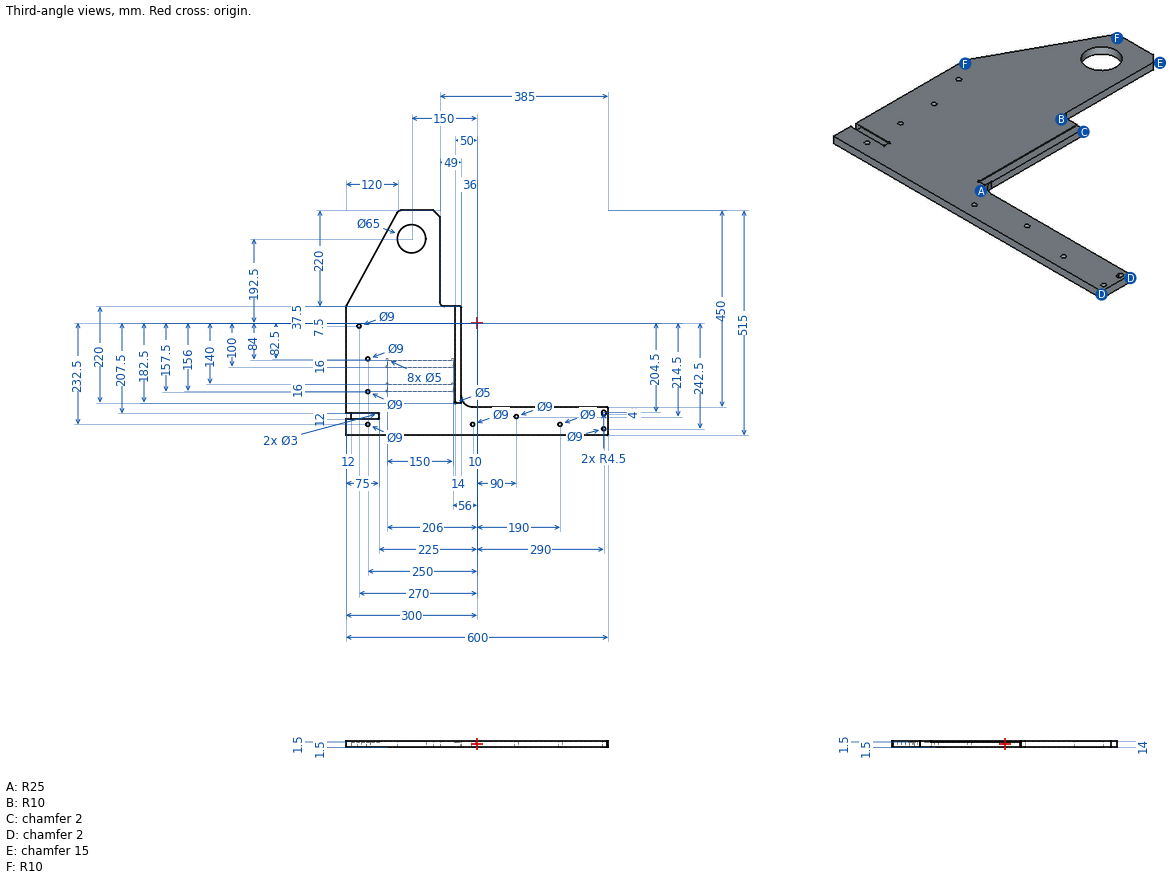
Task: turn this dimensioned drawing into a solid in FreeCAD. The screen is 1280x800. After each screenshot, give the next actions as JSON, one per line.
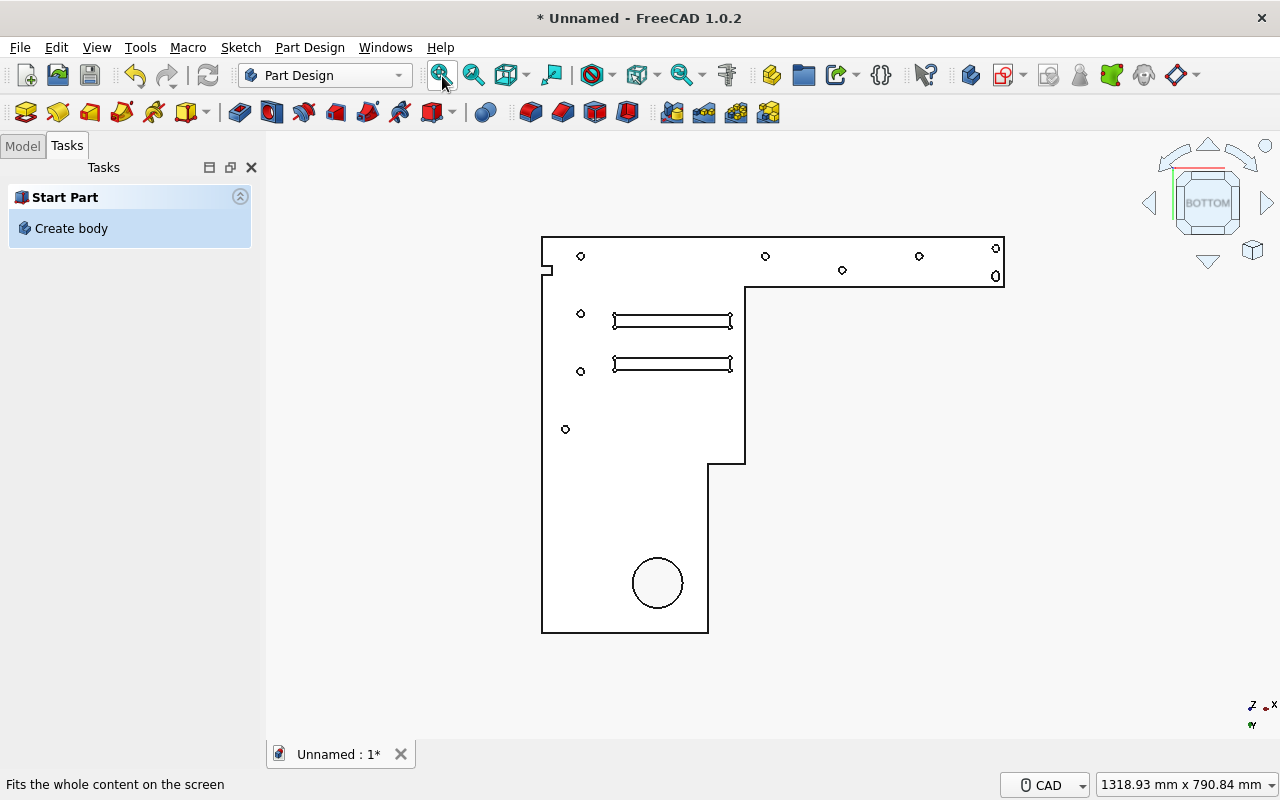
{"action": "key", "text": "4"}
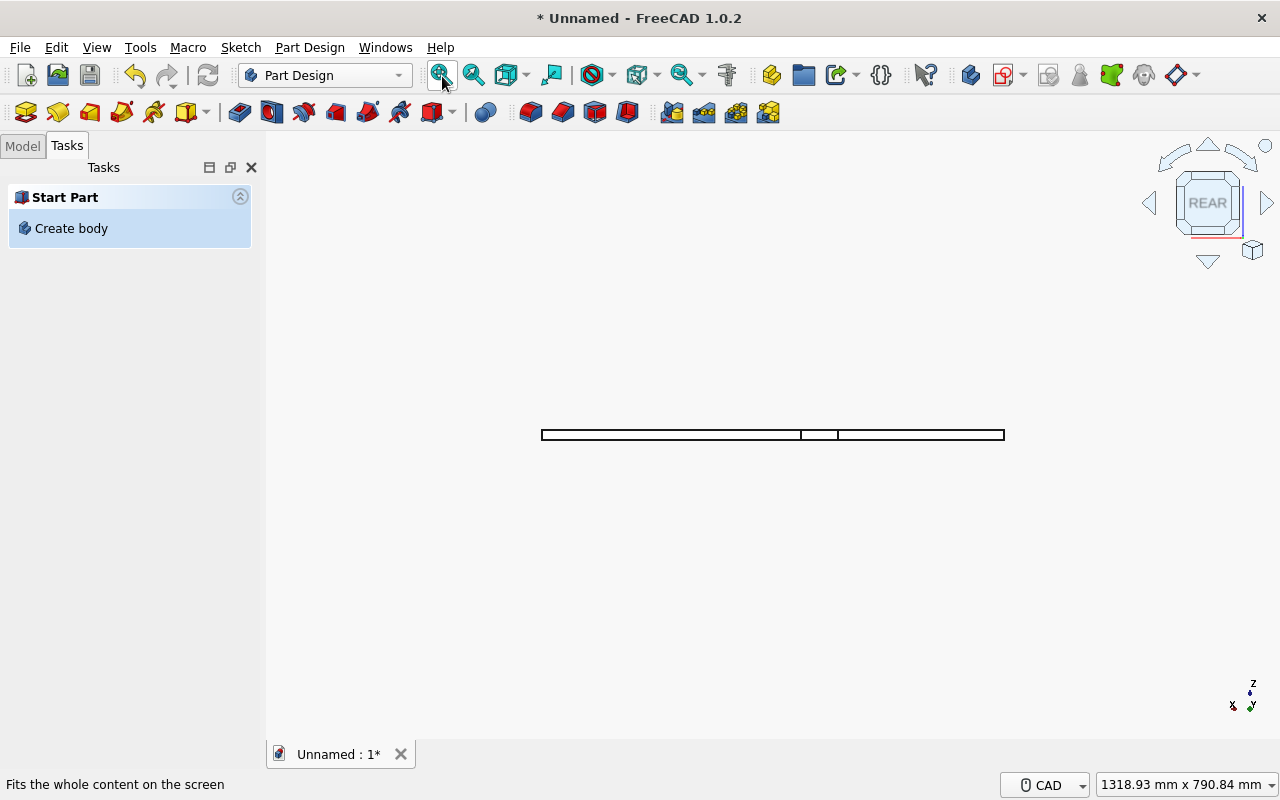
{"action": "scroll", "coordinate": [801, 434], "scroll_direction": "up", "scroll_amount": 7}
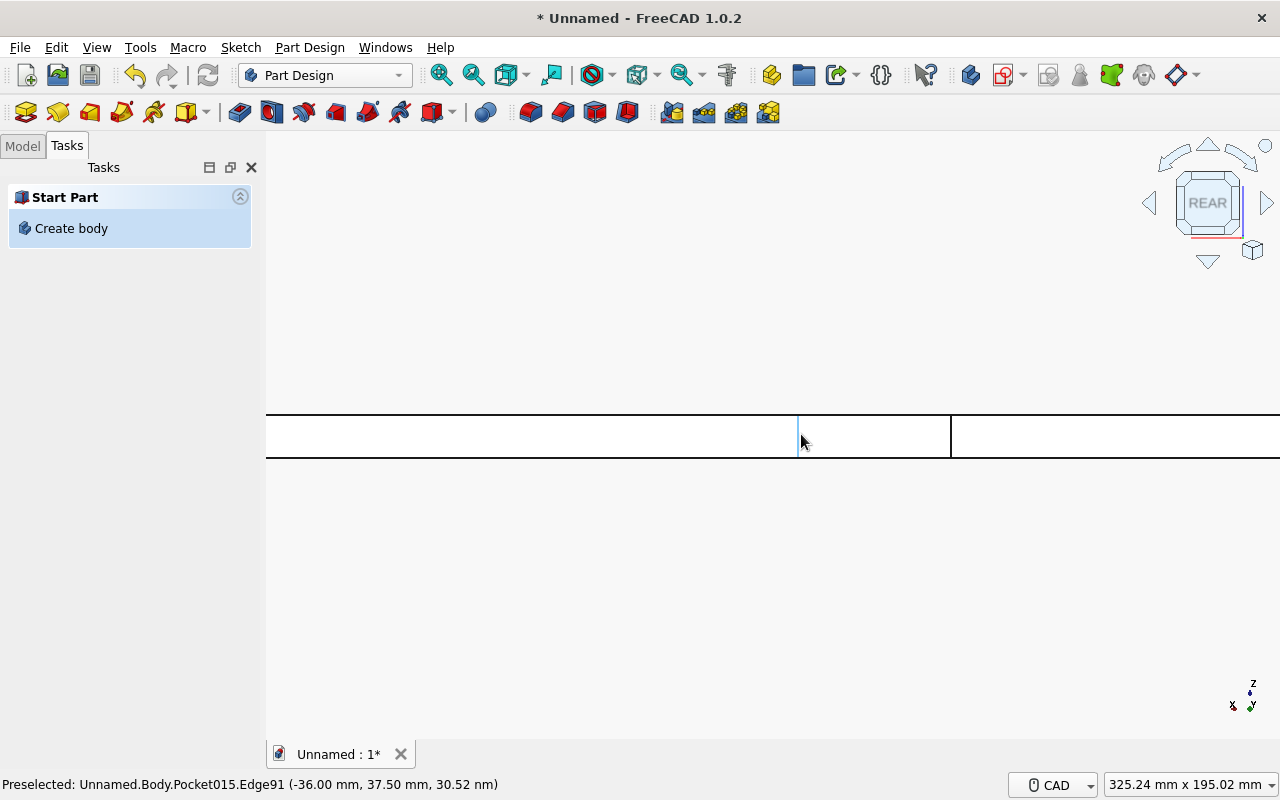
{"action": "left_click", "coordinate": [442, 76]}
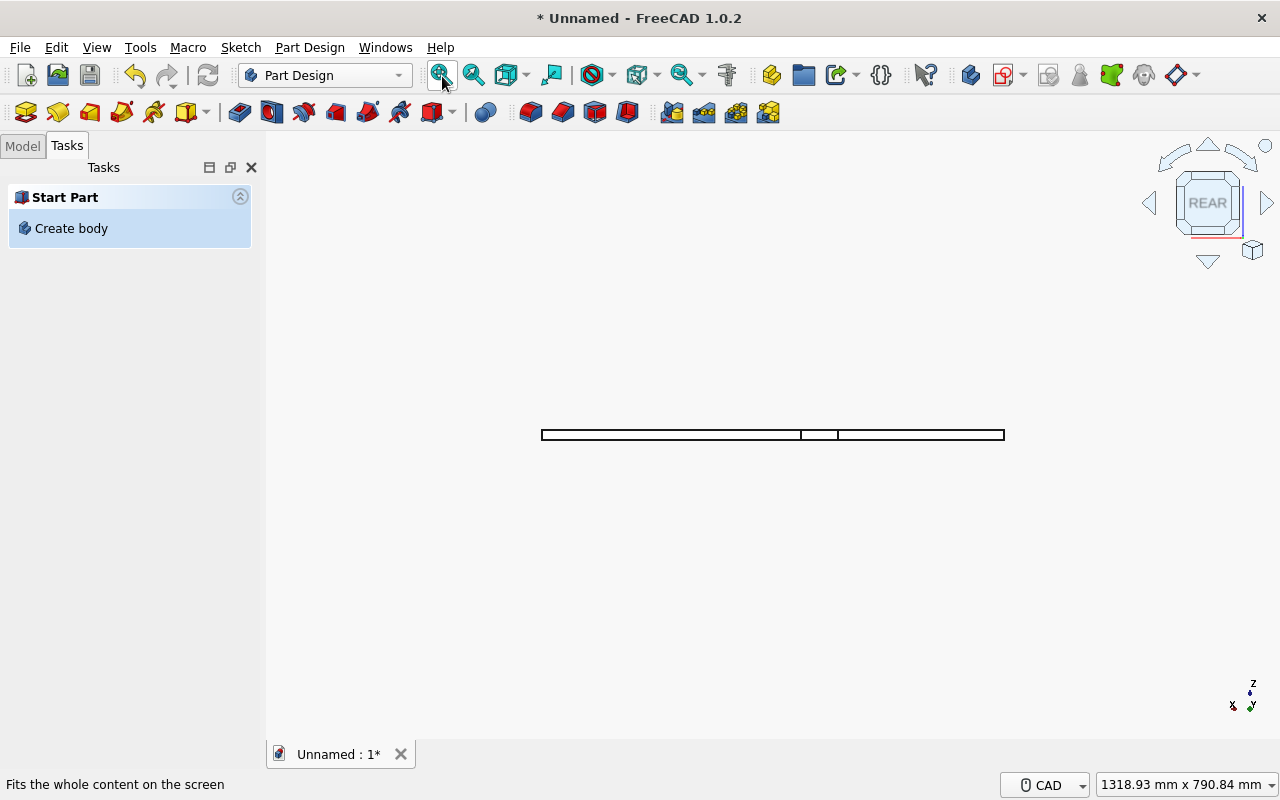
{"action": "key", "text": "6"}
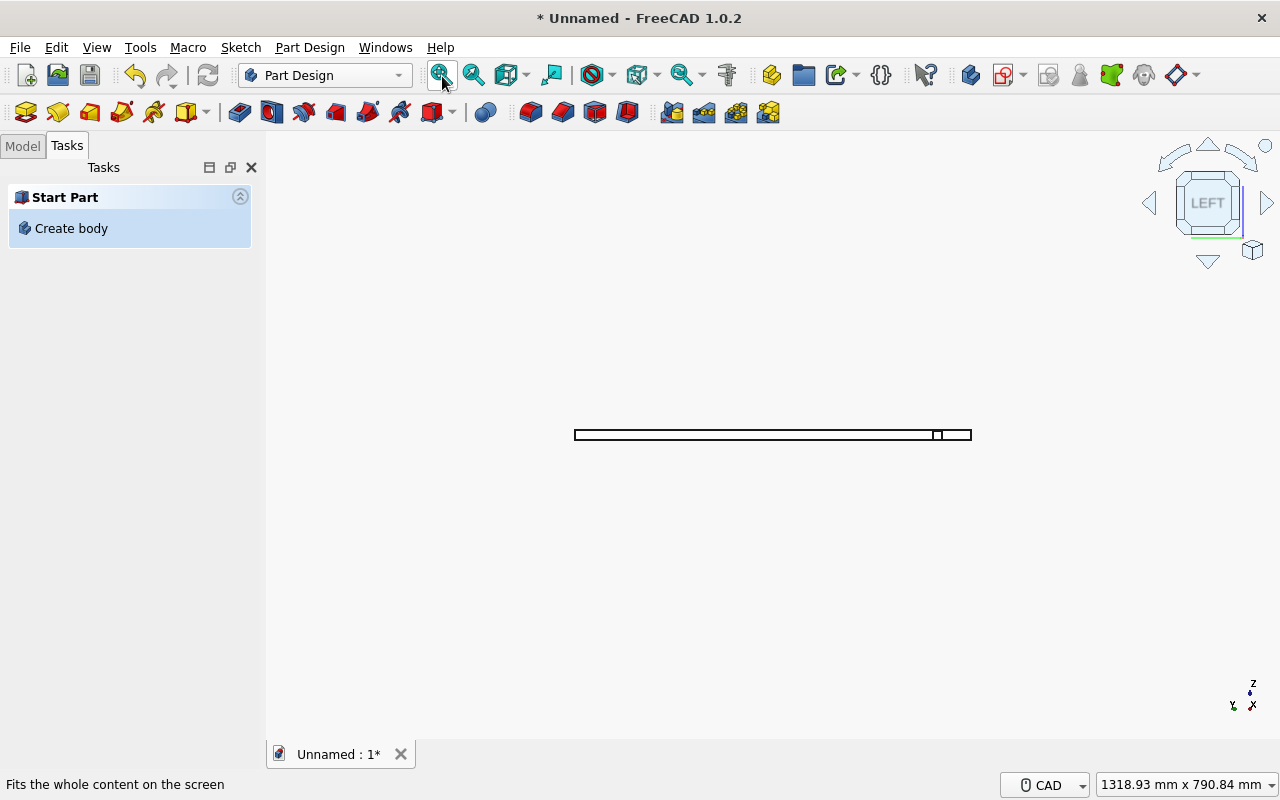
{"action": "left_click", "coordinate": [442, 76]}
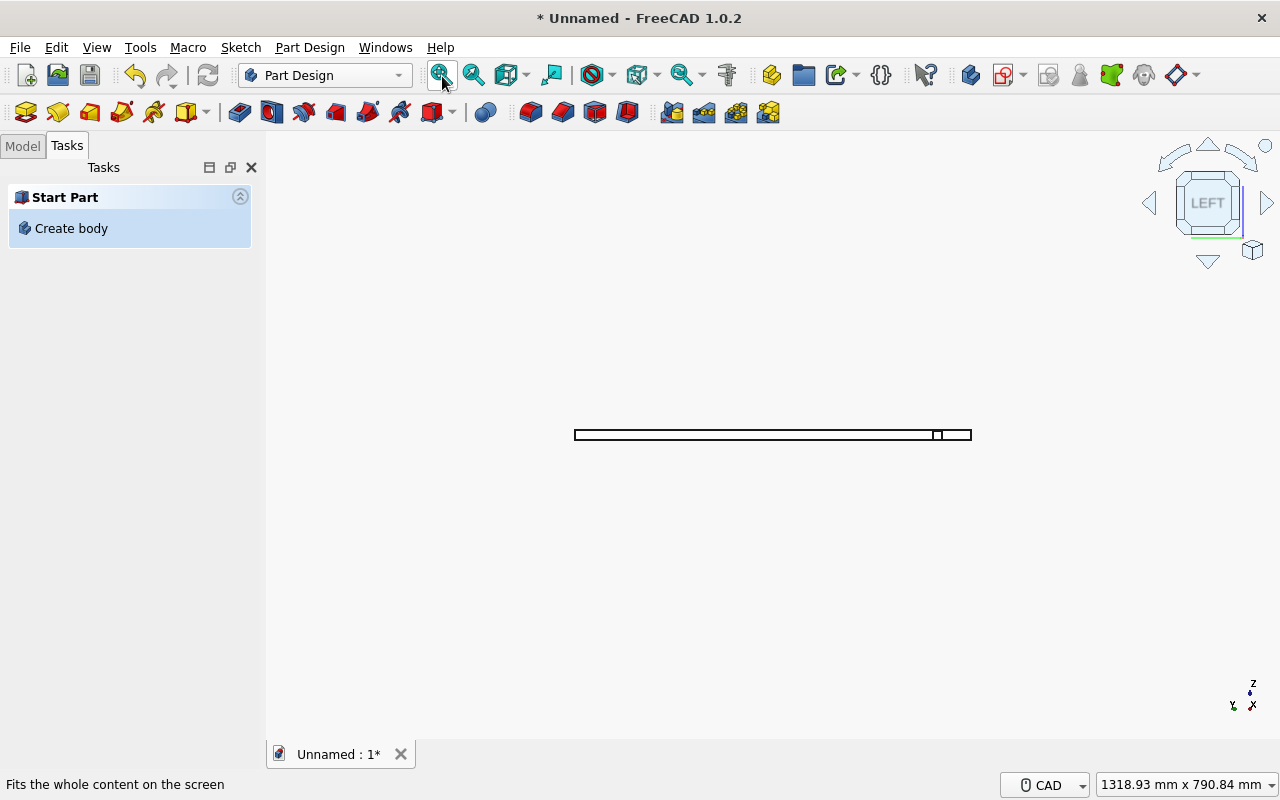
{"action": "scroll", "coordinate": [921, 434], "scroll_direction": "up", "scroll_amount": 7}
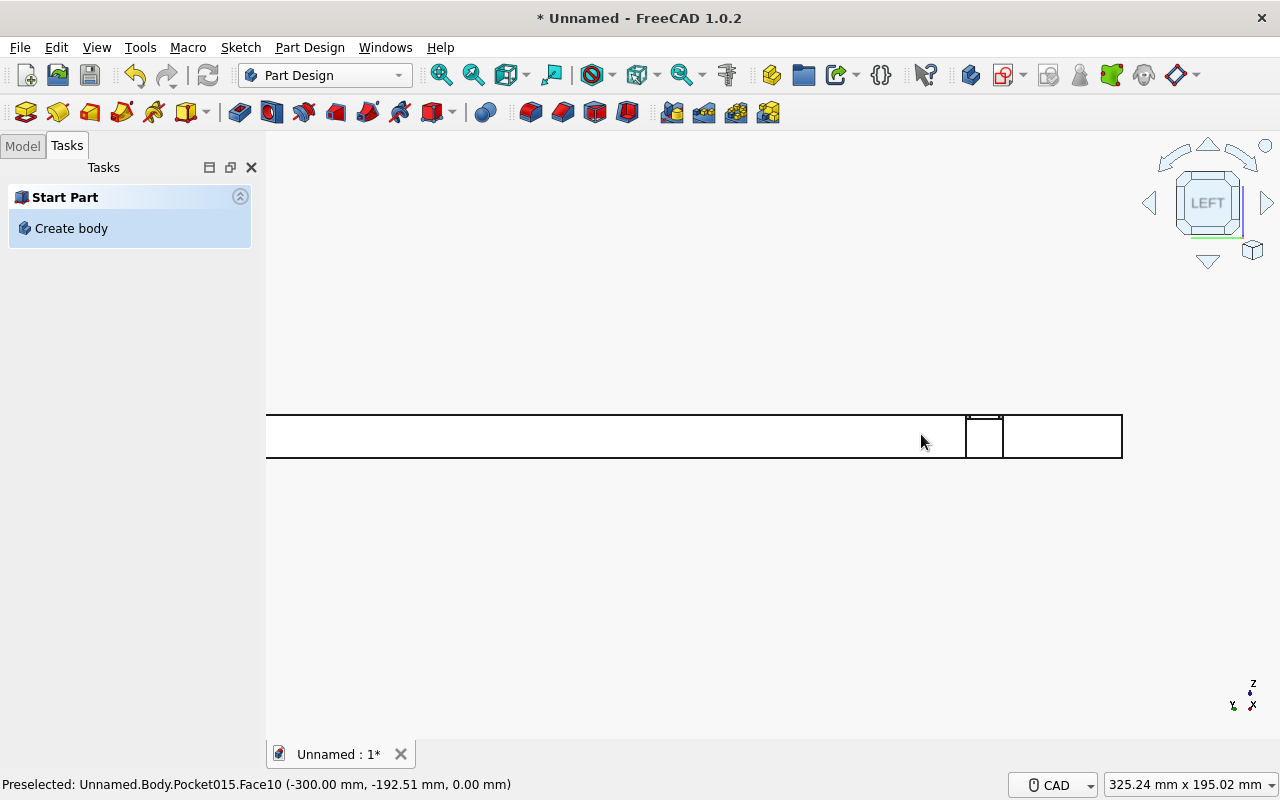
{"action": "left_click", "coordinate": [442, 76]}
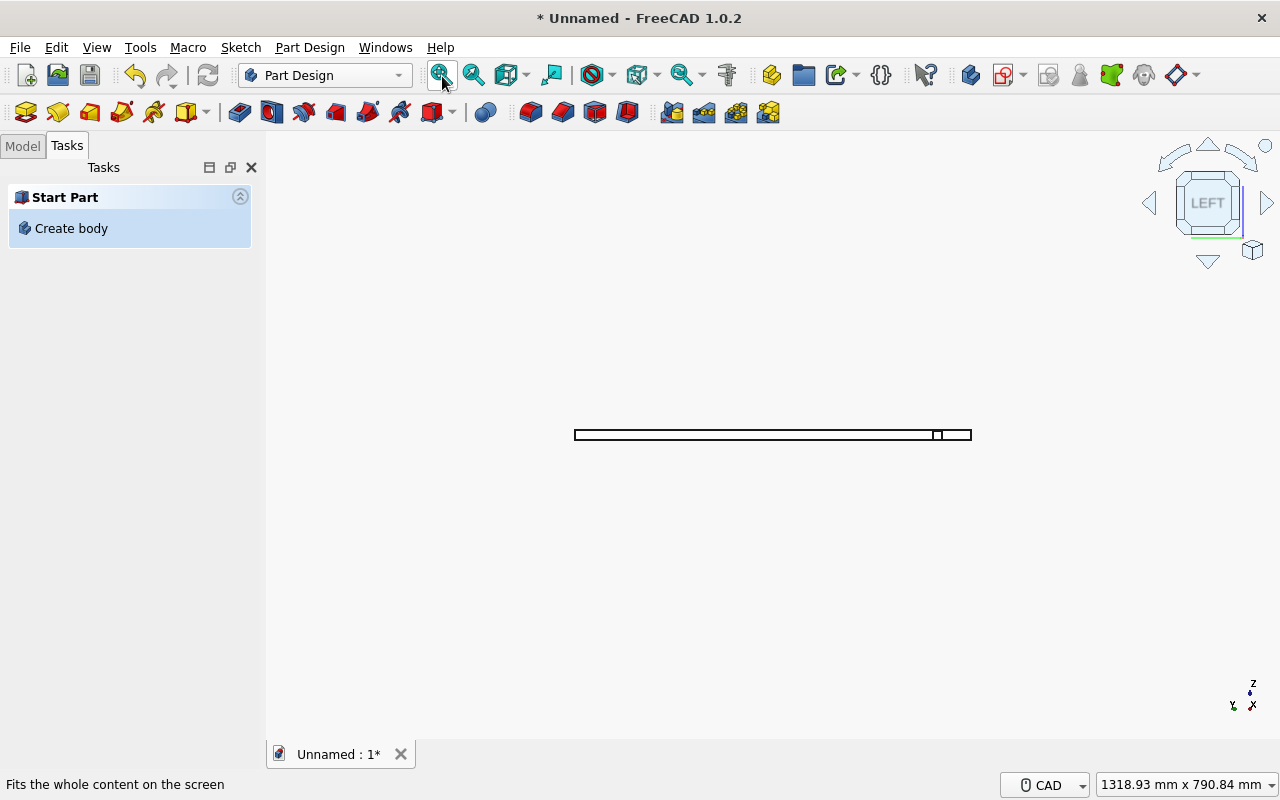
{"action": "key", "text": "v 3"}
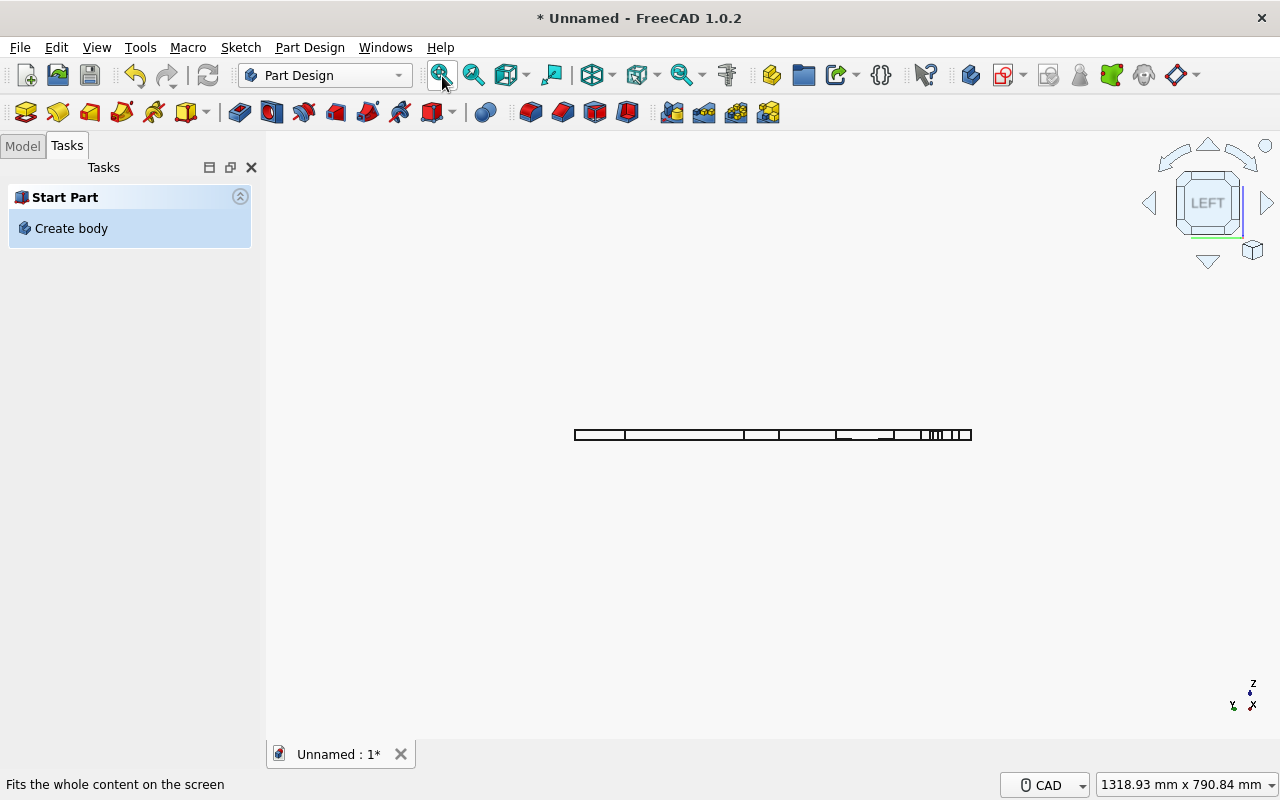
{"action": "key", "text": "0"}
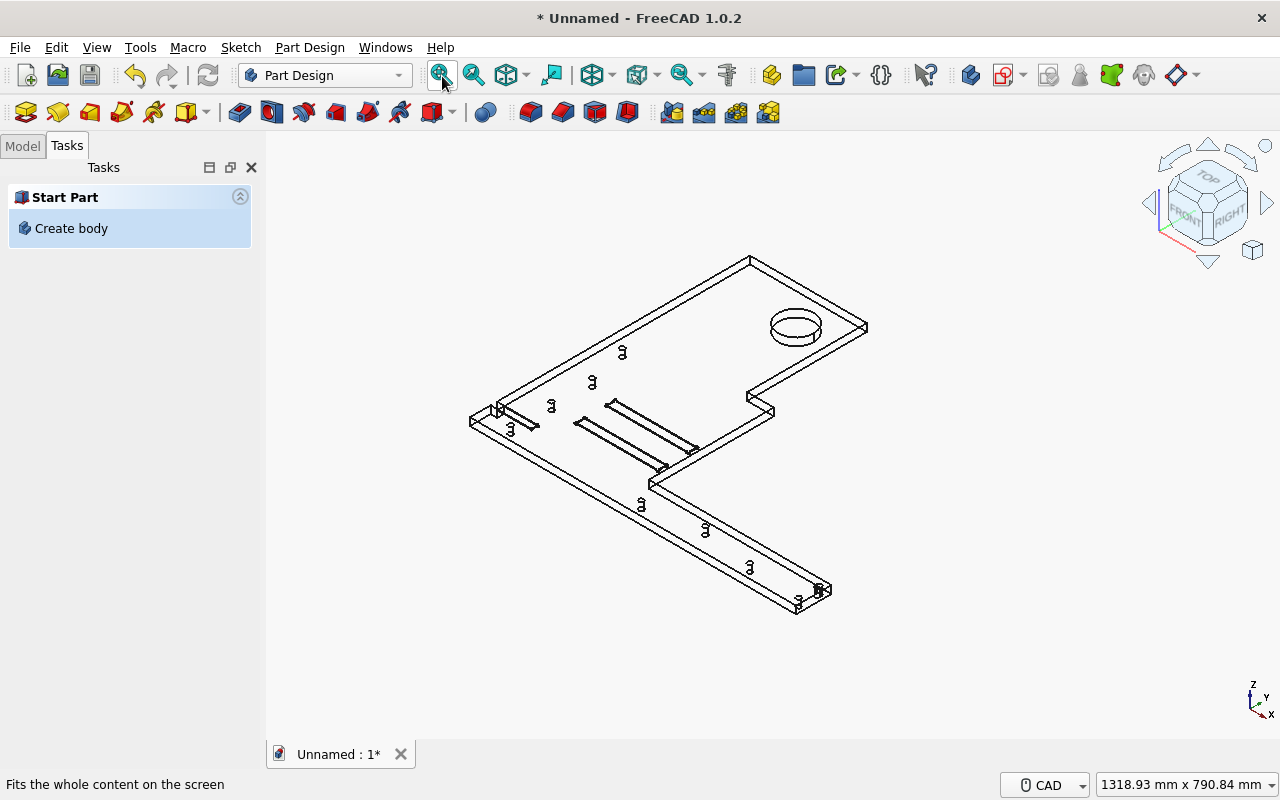
{"action": "scroll", "coordinate": [649, 483], "scroll_direction": "up", "scroll_amount": 7}